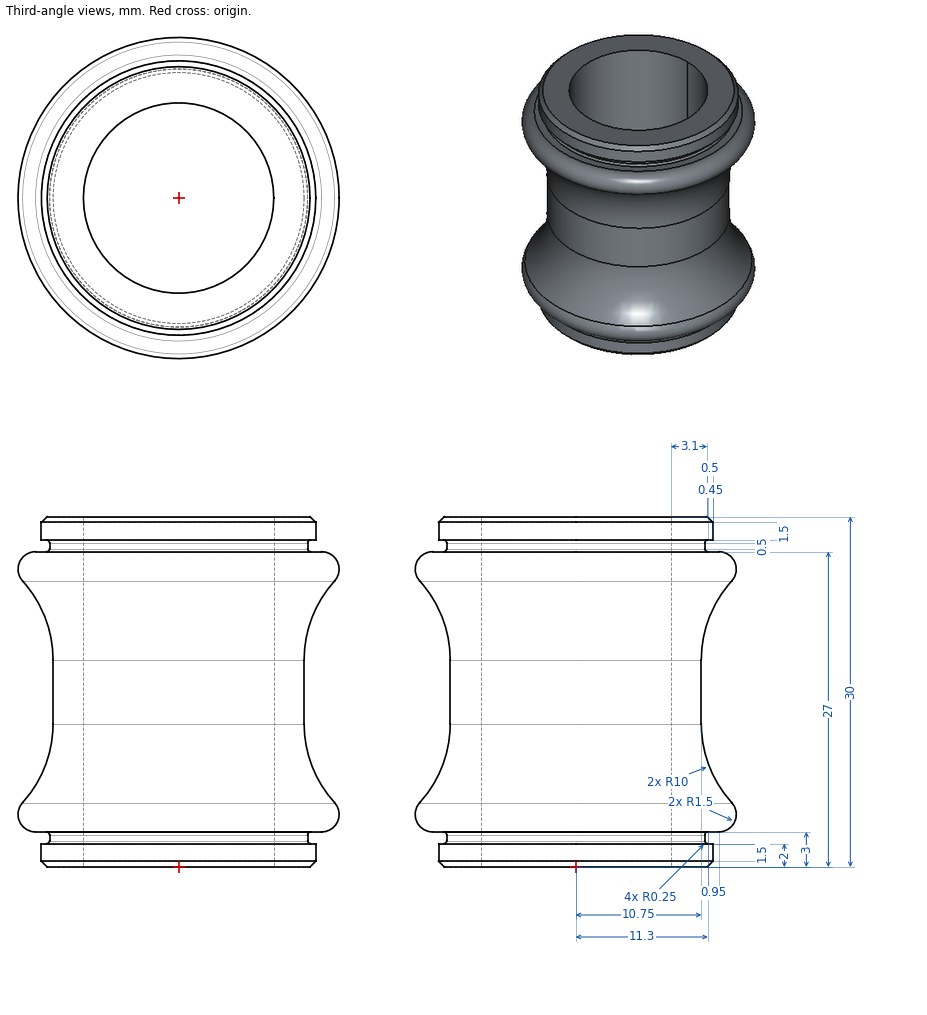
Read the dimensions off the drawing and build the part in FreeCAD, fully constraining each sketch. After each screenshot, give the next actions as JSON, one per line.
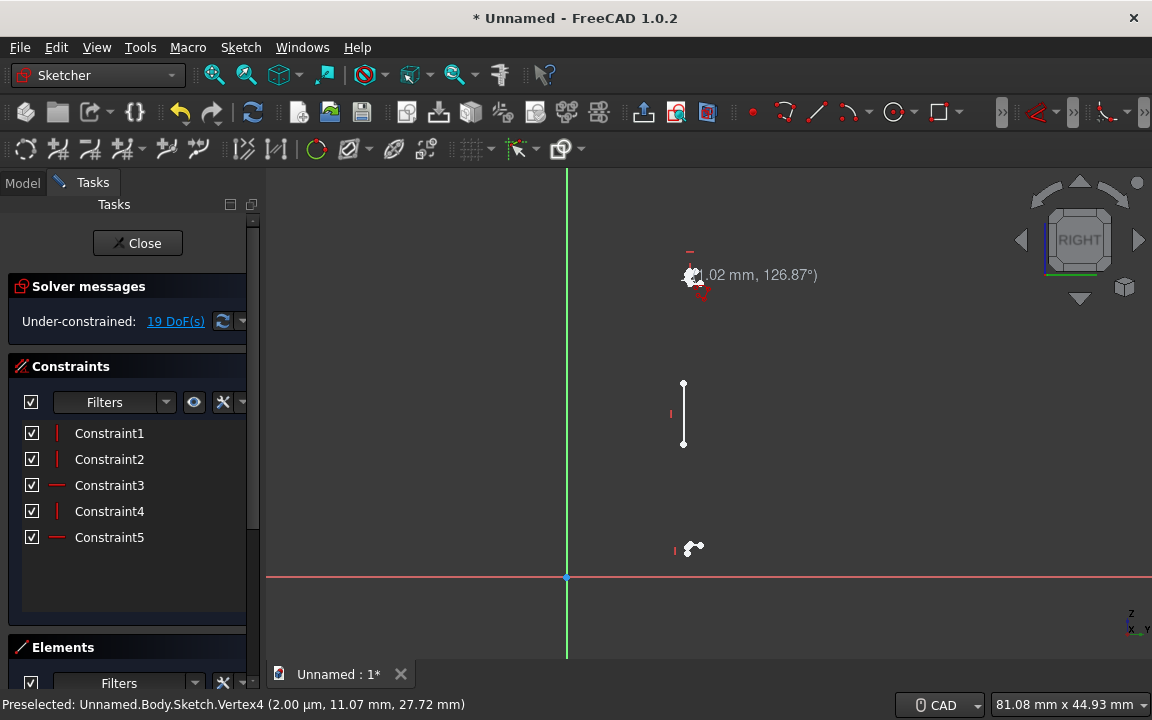
{"action": "left_click", "coordinate": [695, 255]}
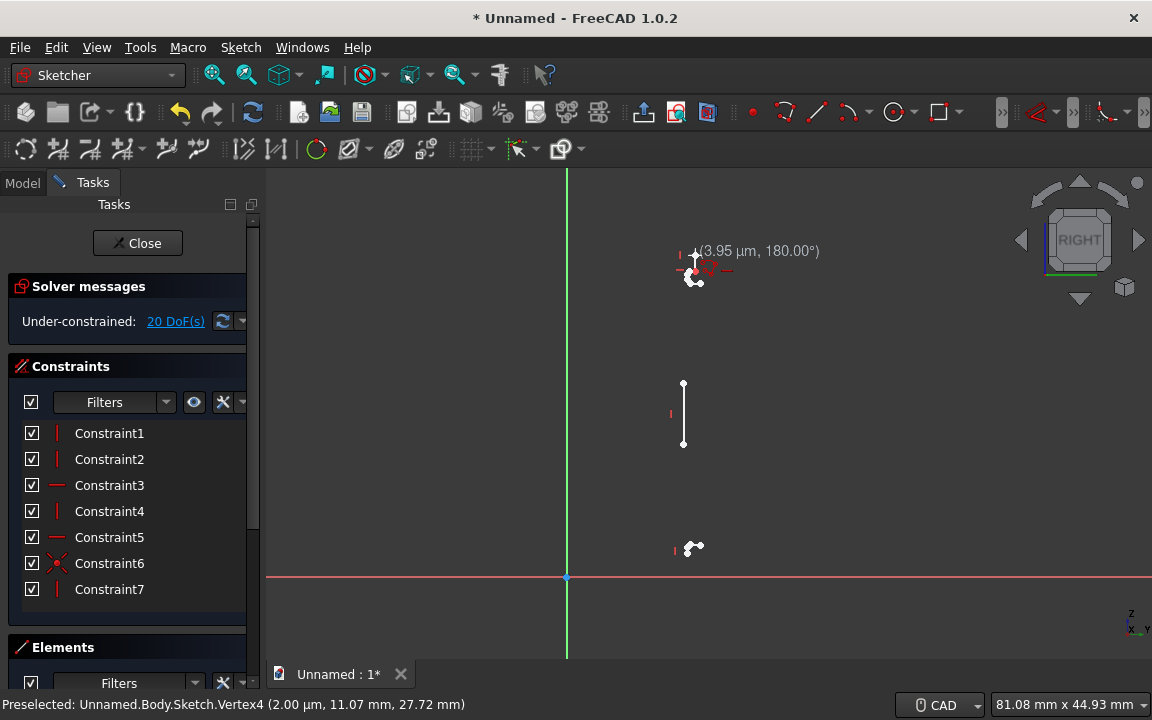
{"action": "scroll", "coordinate": [690, 249], "scroll_direction": "up", "scroll_amount": 4}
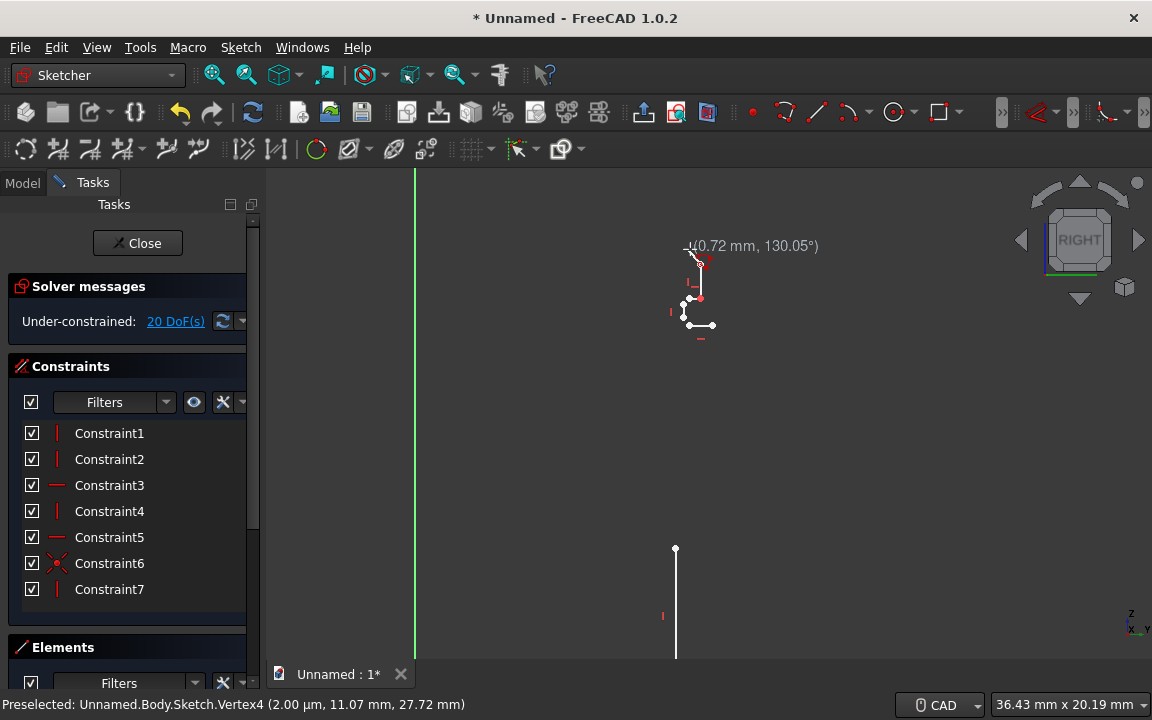
{"action": "left_click", "coordinate": [688, 250]}
{"action": "left_click", "coordinate": [613, 250]}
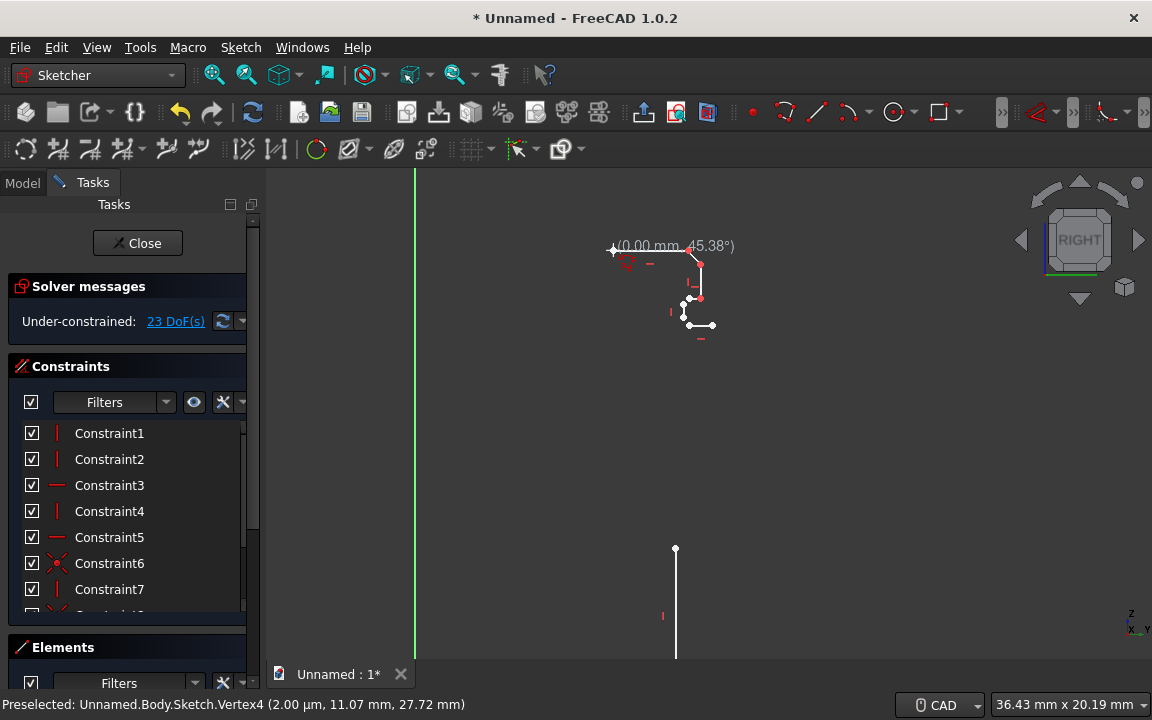
{"action": "scroll", "coordinate": [690, 249], "scroll_direction": "down", "scroll_amount": 4}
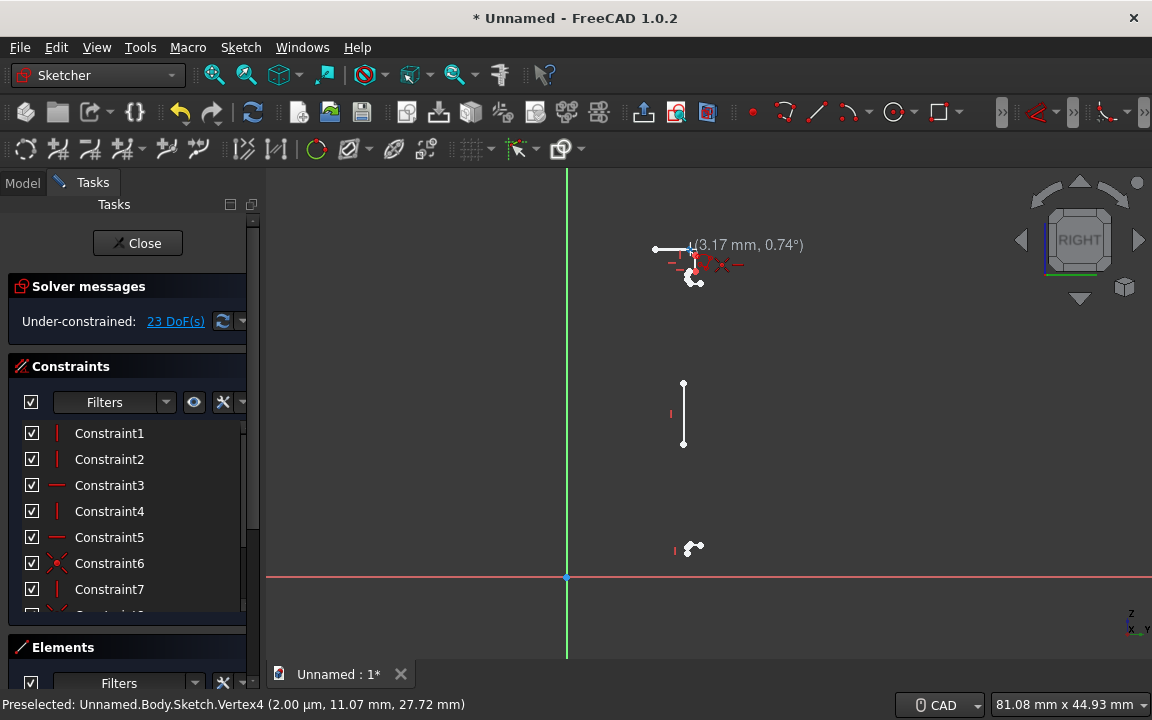
{"action": "left_click", "coordinate": [656, 577]}
{"action": "left_click", "coordinate": [690, 568]}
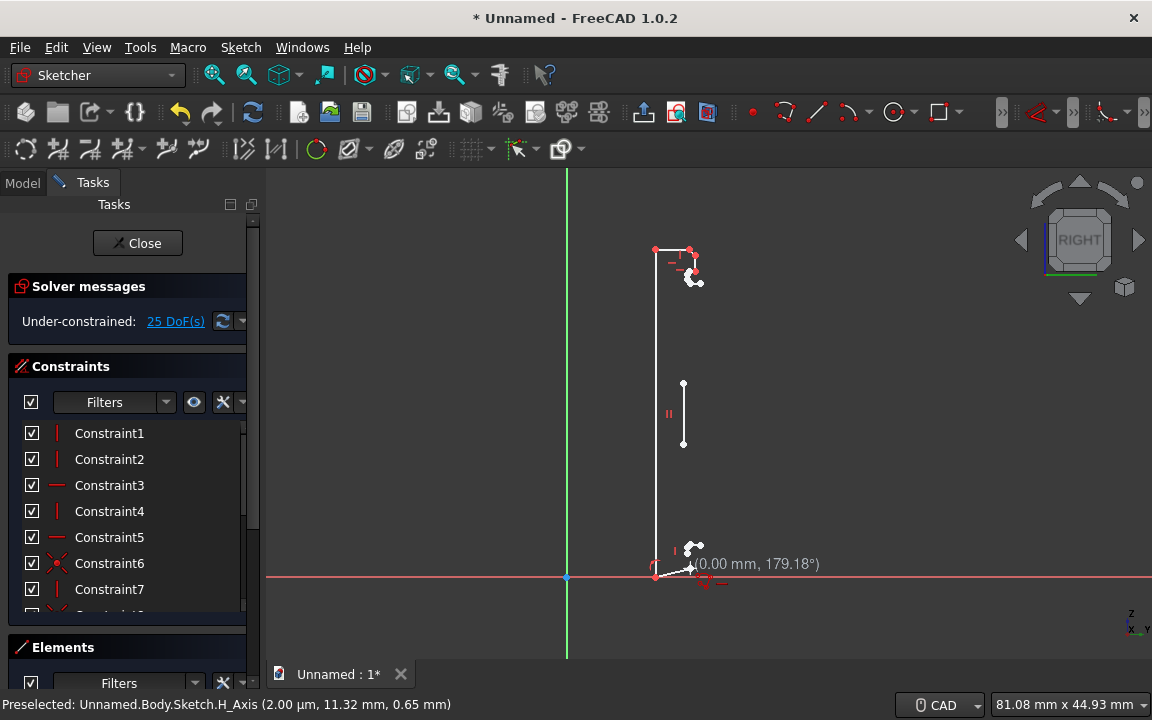
{"action": "scroll", "coordinate": [695, 572], "scroll_direction": "up", "scroll_amount": 6}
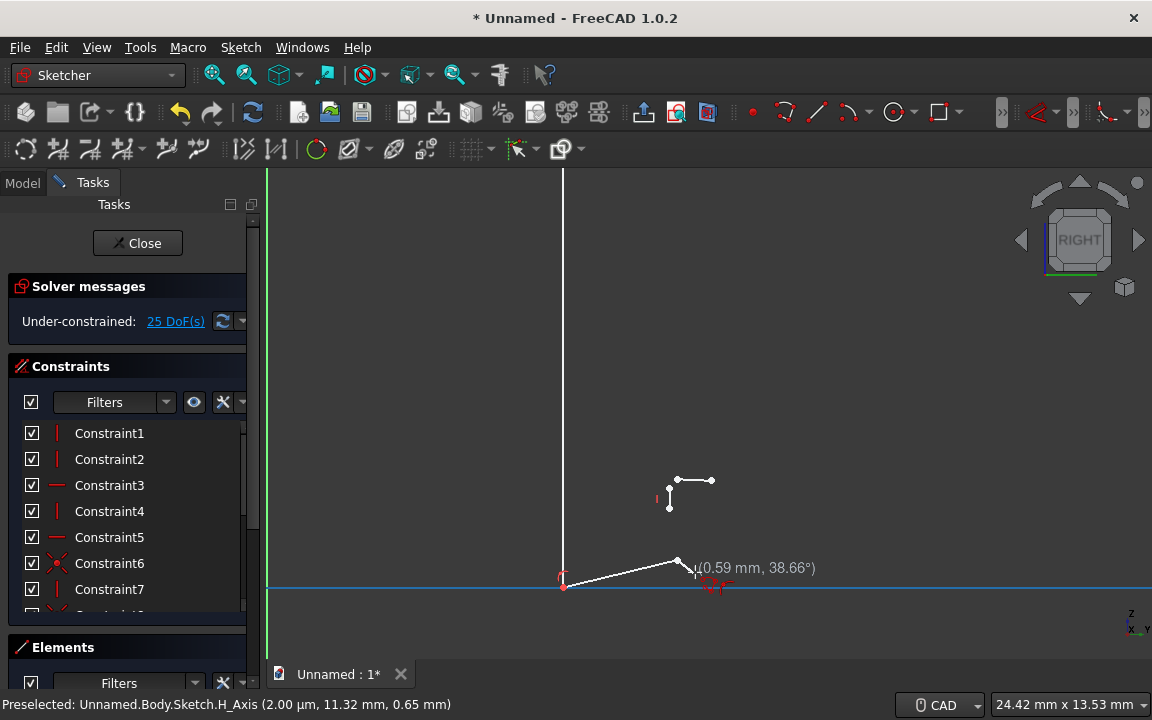
{"action": "left_click", "coordinate": [694, 569]}
{"action": "left_click", "coordinate": [694, 515]}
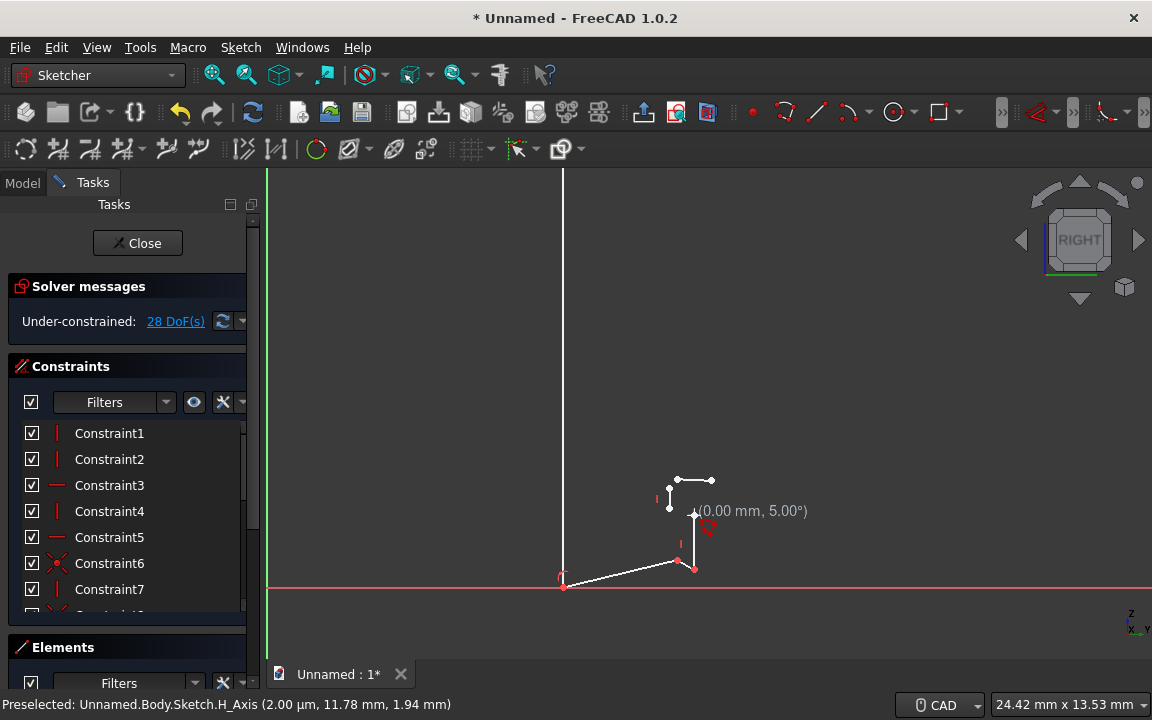
{"action": "scroll", "coordinate": [677, 515], "scroll_direction": "up", "scroll_amount": 2}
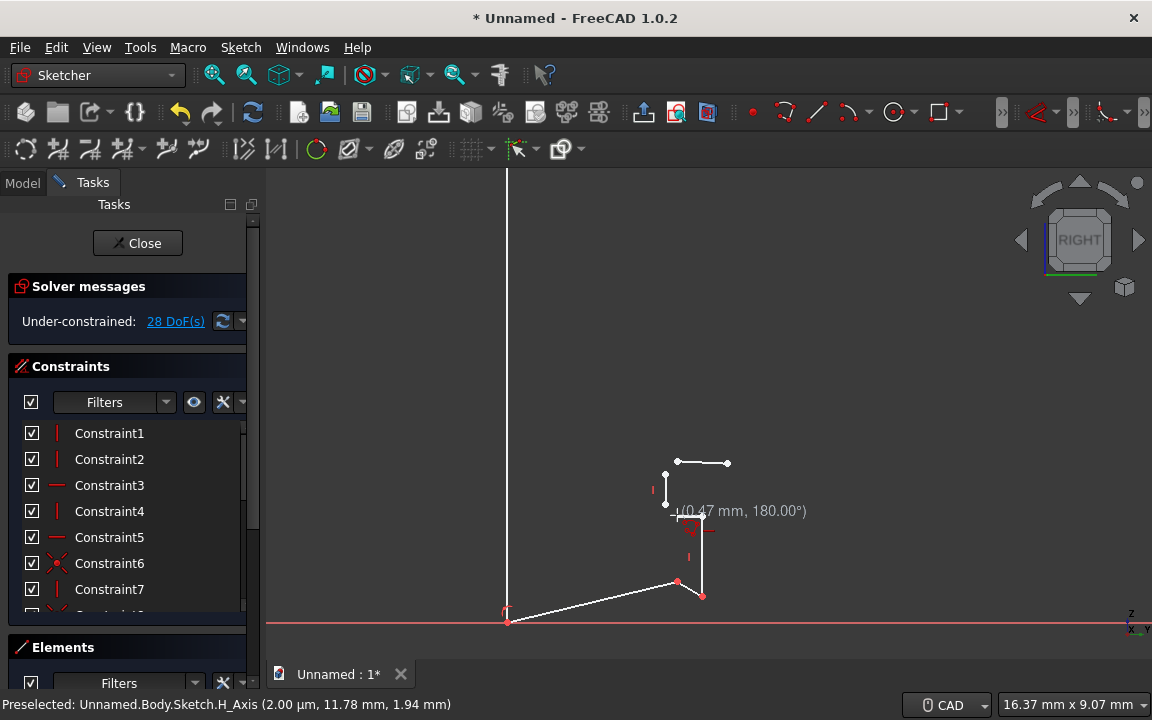
{"action": "left_click", "coordinate": [677, 515]}
{"action": "right_click", "coordinate": [677, 515]}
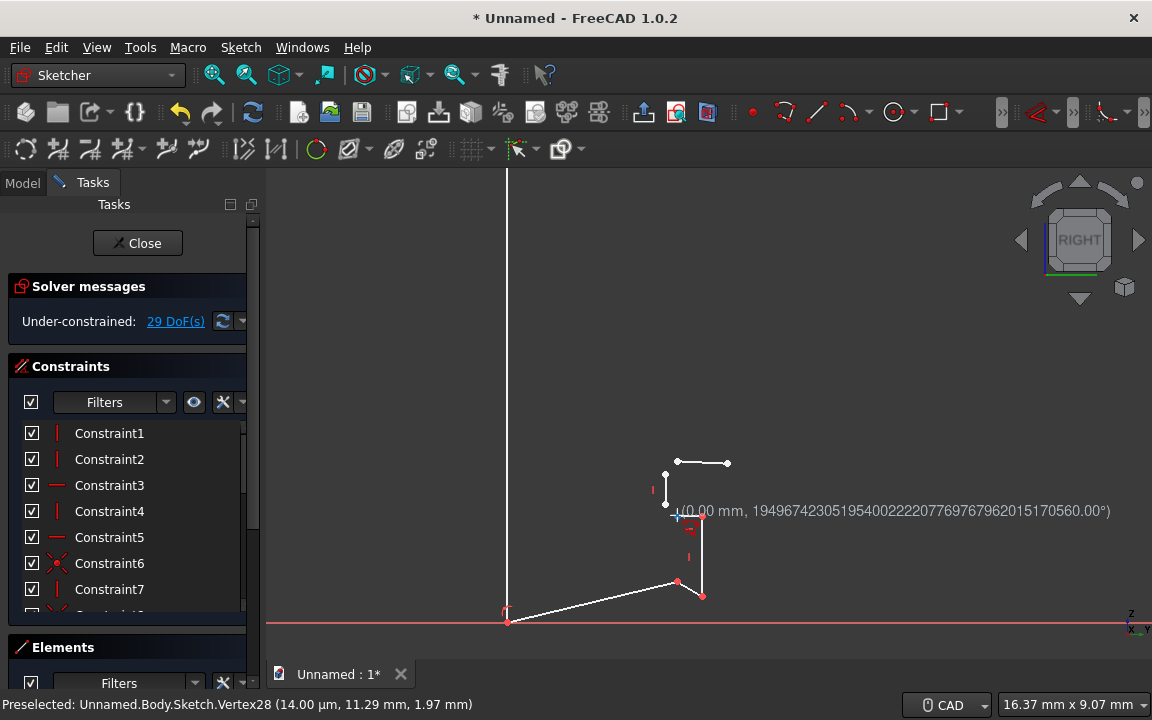
{"action": "left_click", "coordinate": [872, 112]}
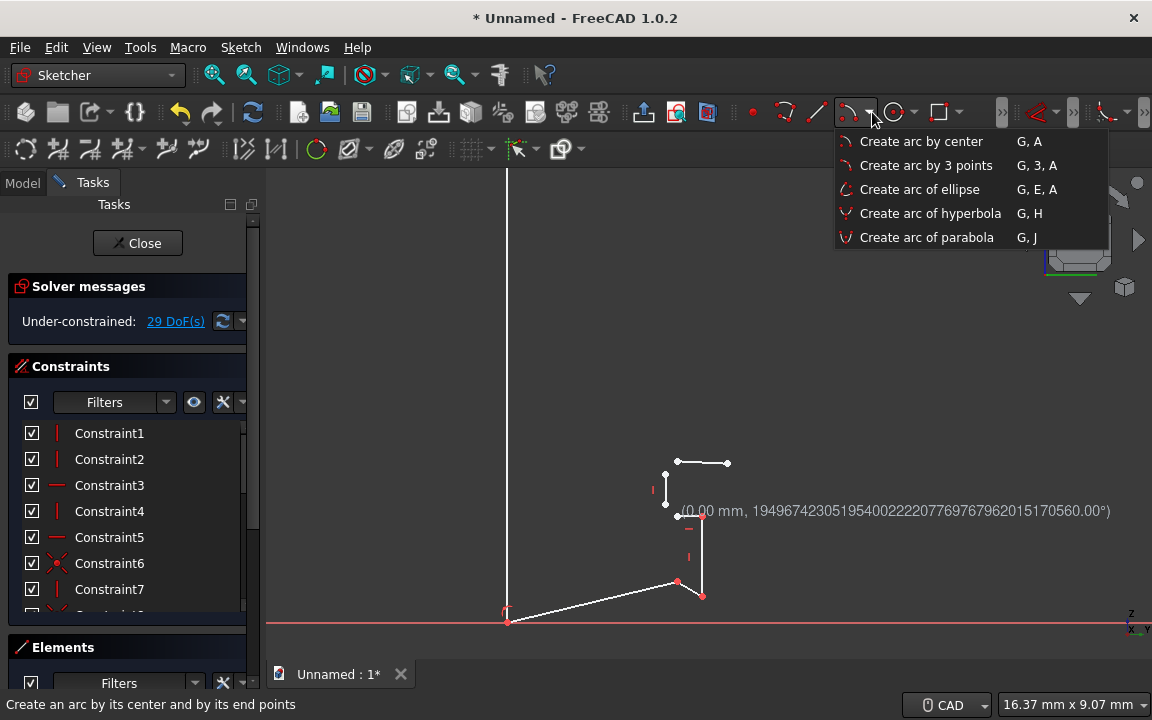
{"action": "left_click", "coordinate": [972, 165]}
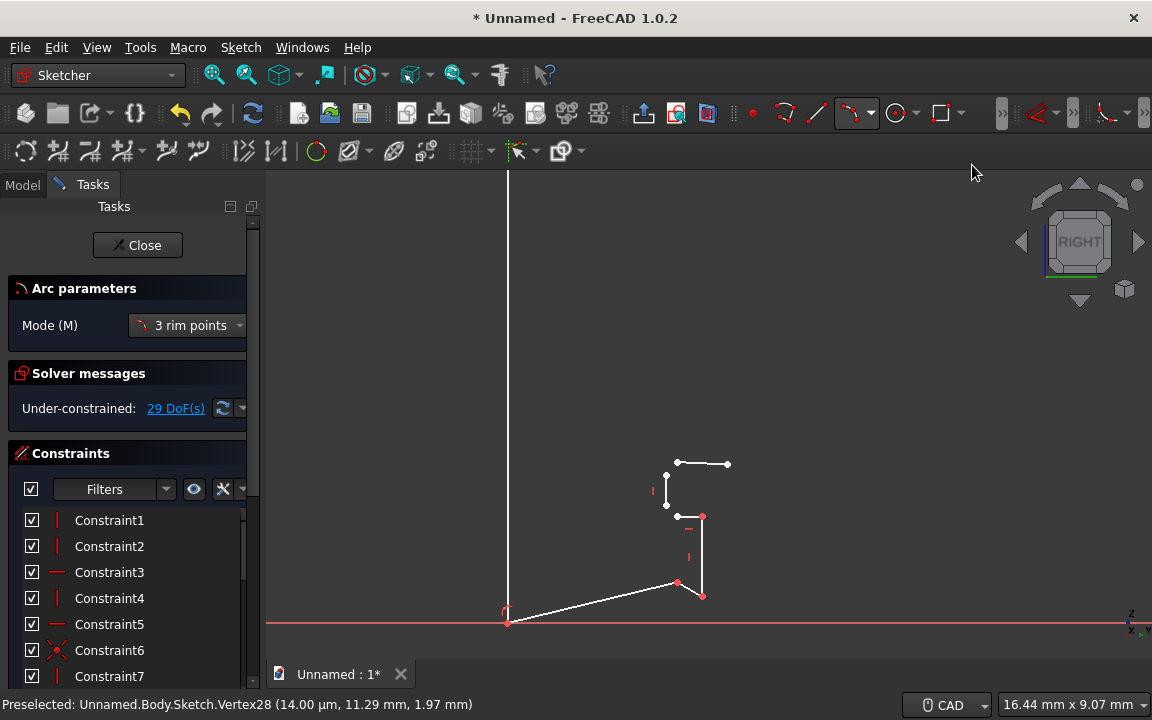
{"action": "left_click", "coordinate": [666, 476]}
{"action": "left_click", "coordinate": [677, 462]}